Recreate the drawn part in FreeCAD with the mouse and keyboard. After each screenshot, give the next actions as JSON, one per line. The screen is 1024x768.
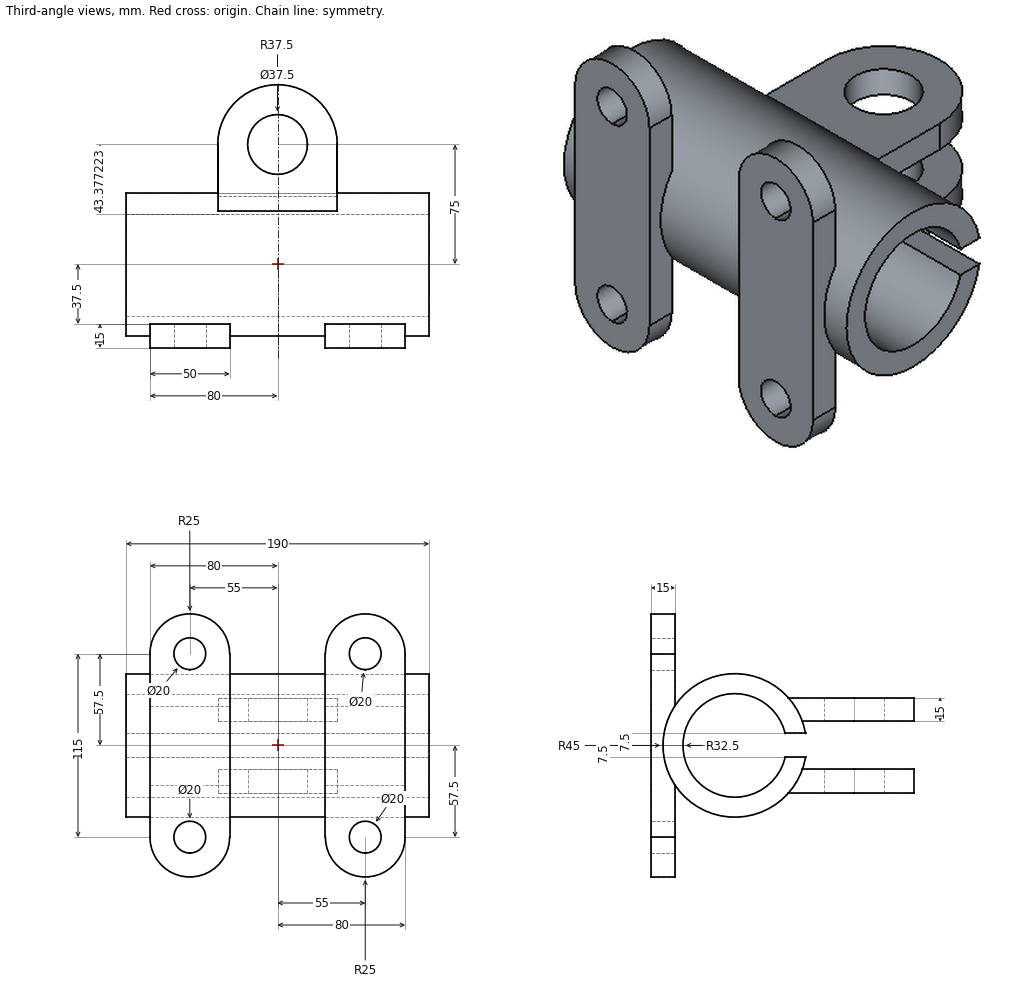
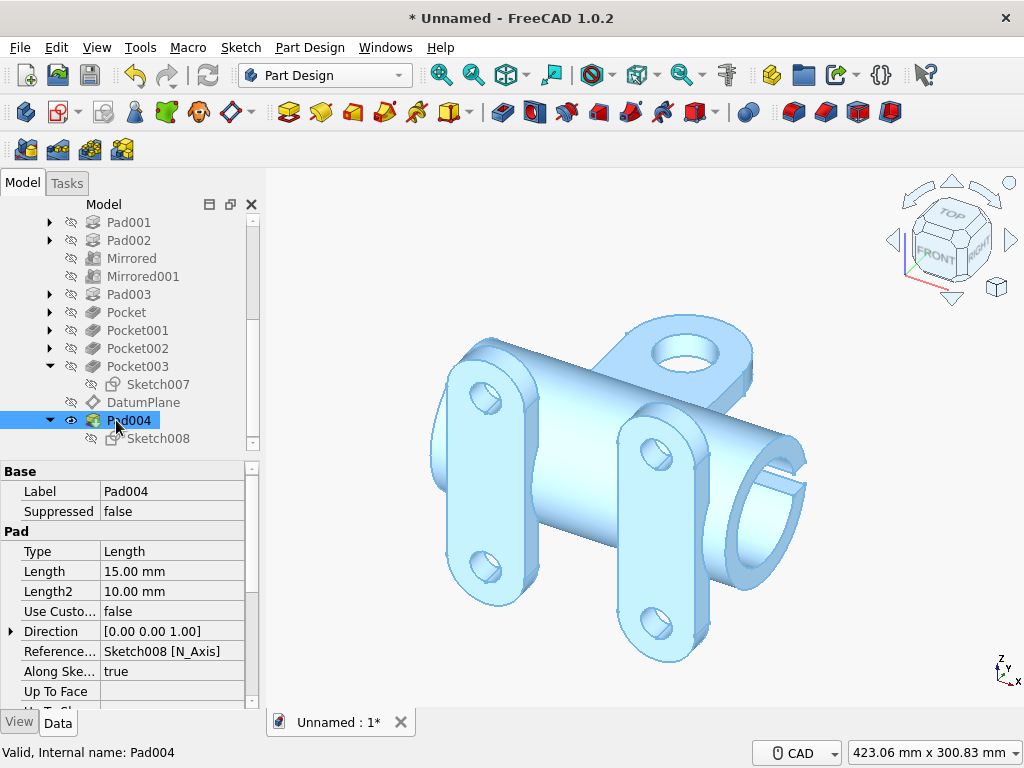
{"action": "left_click", "coordinate": [26, 150]}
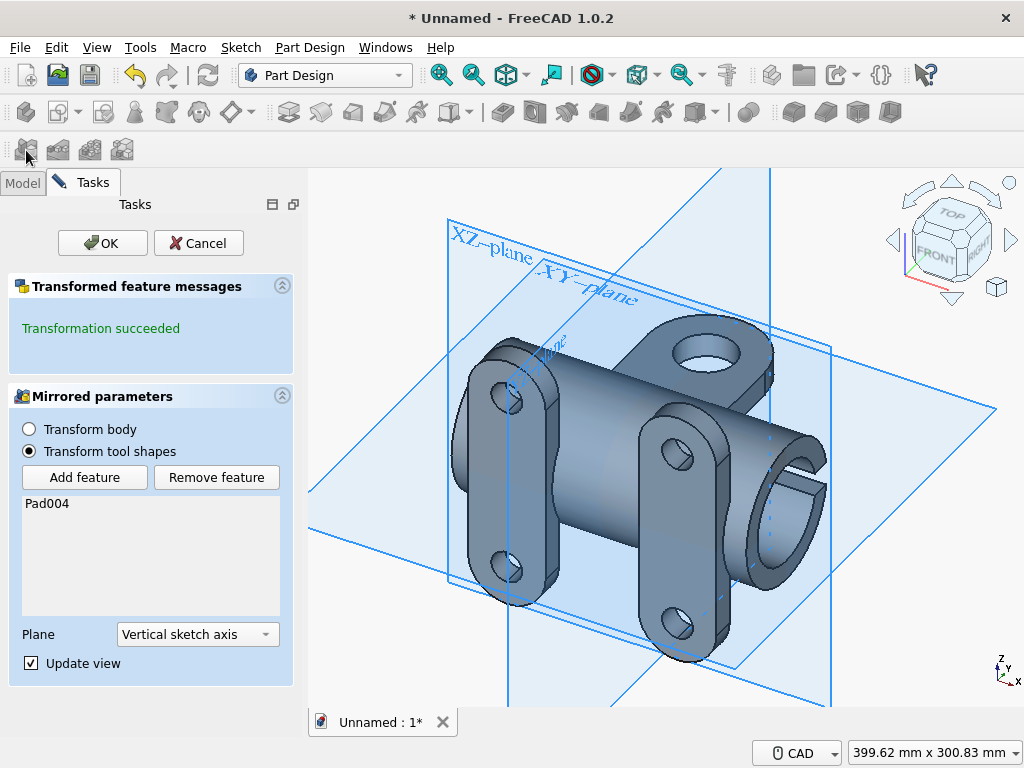
{"action": "left_click", "coordinate": [198, 634]}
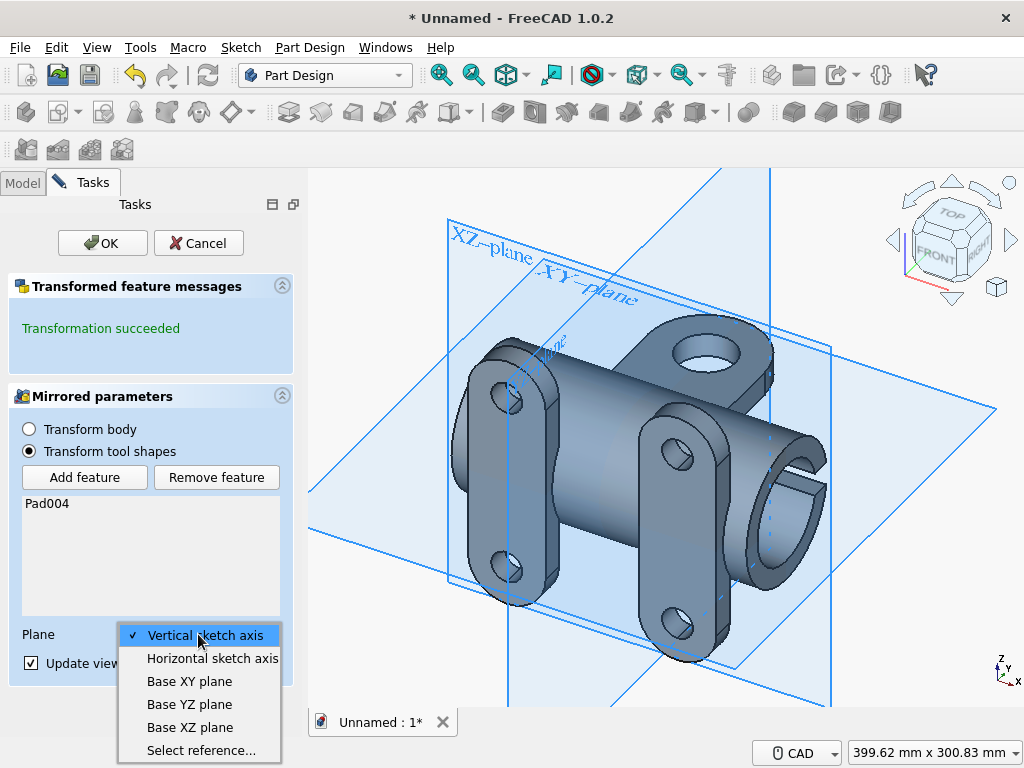
{"action": "left_click", "coordinate": [198, 682]}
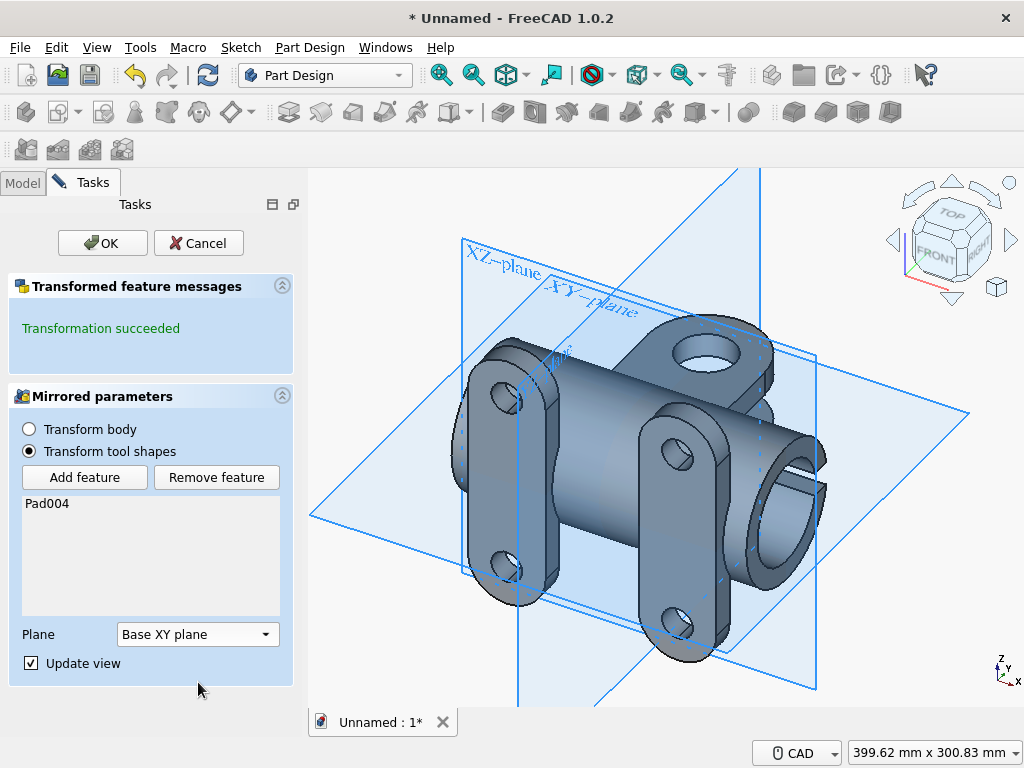
{"action": "left_click", "coordinate": [103, 243]}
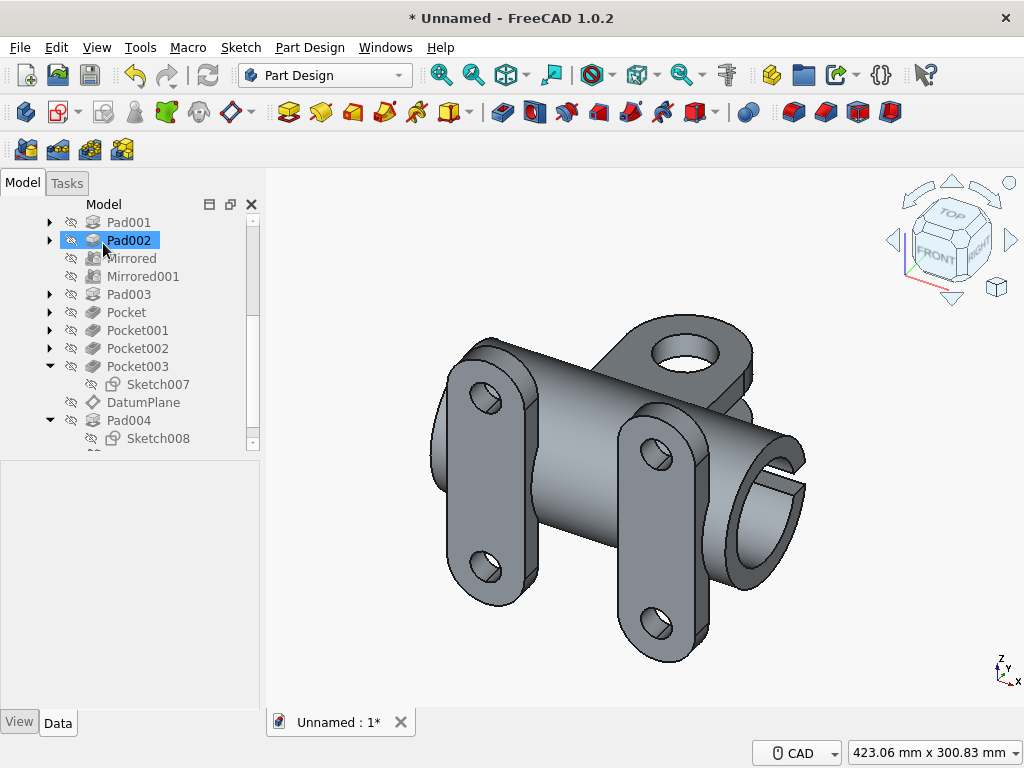
{"action": "key", "text": "0"}